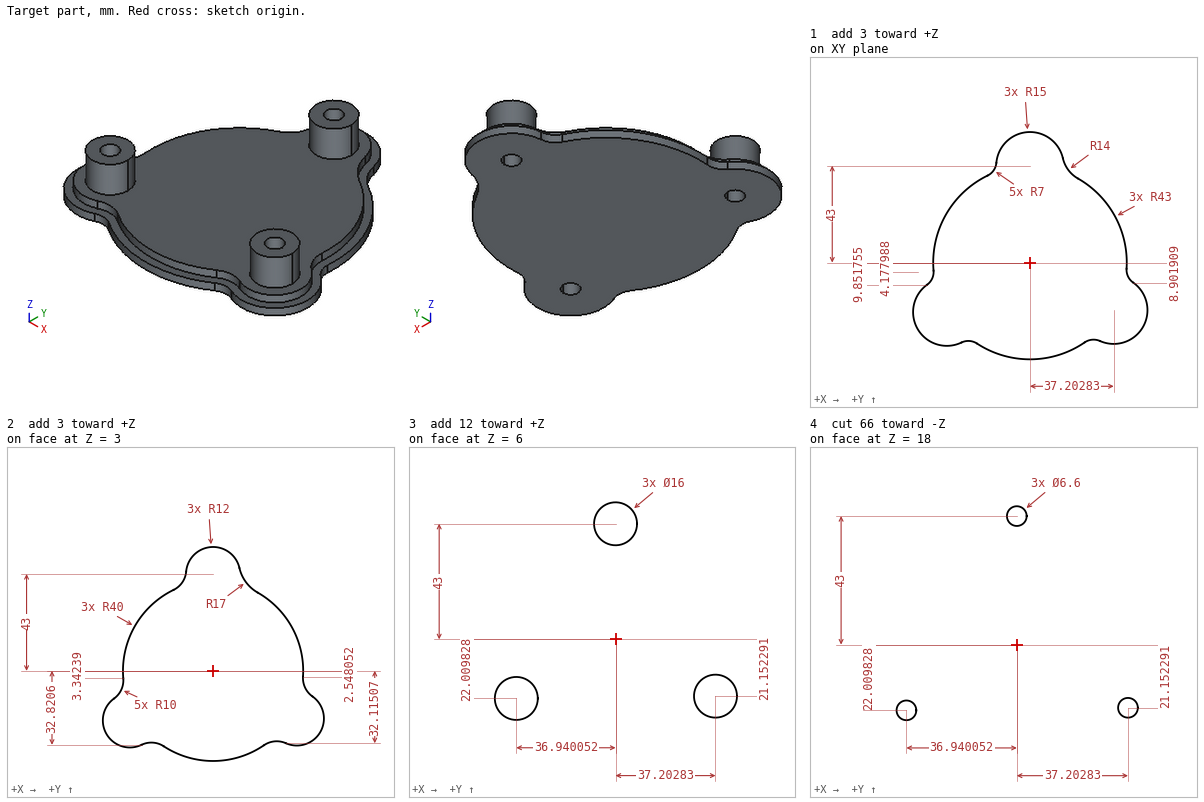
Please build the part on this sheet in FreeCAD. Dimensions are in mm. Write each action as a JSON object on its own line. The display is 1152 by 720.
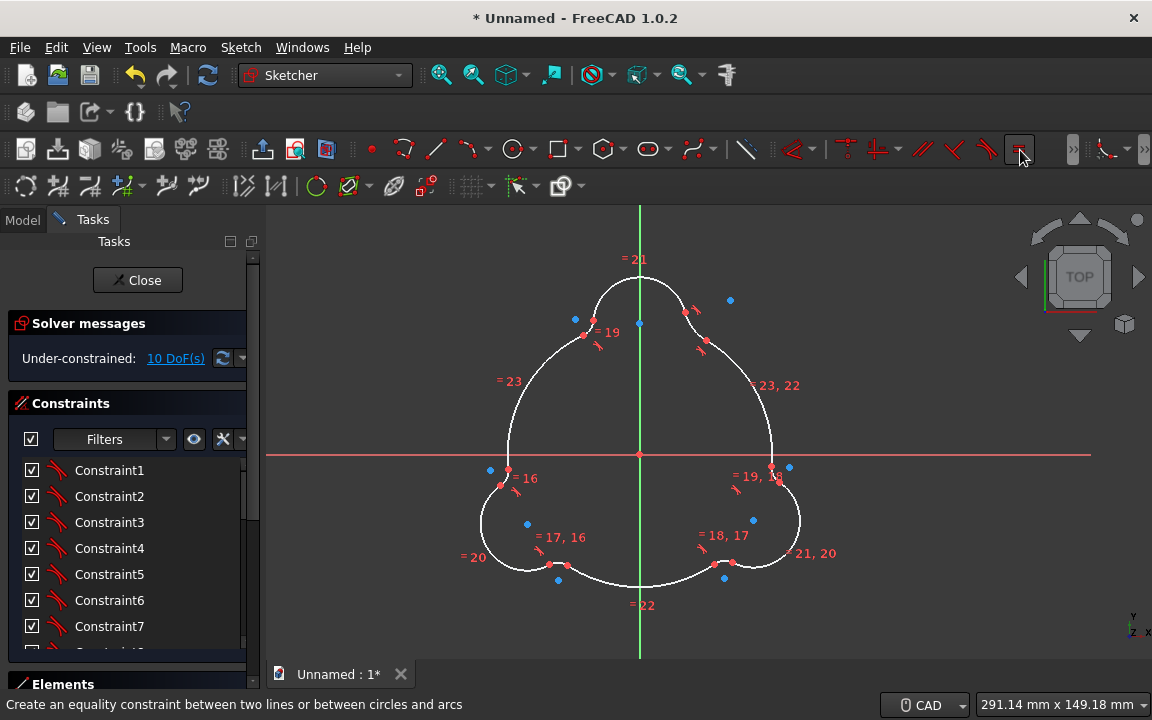
{"action": "left_click", "coordinate": [640, 324]}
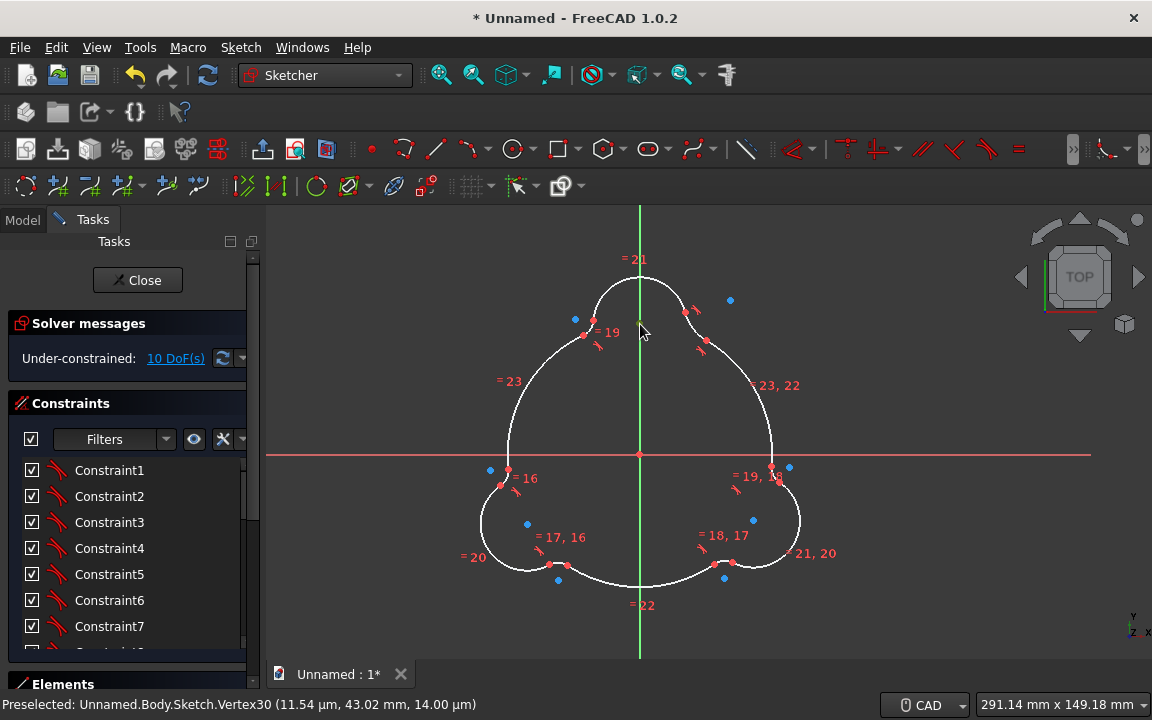
{"action": "left_click", "coordinate": [640, 546]}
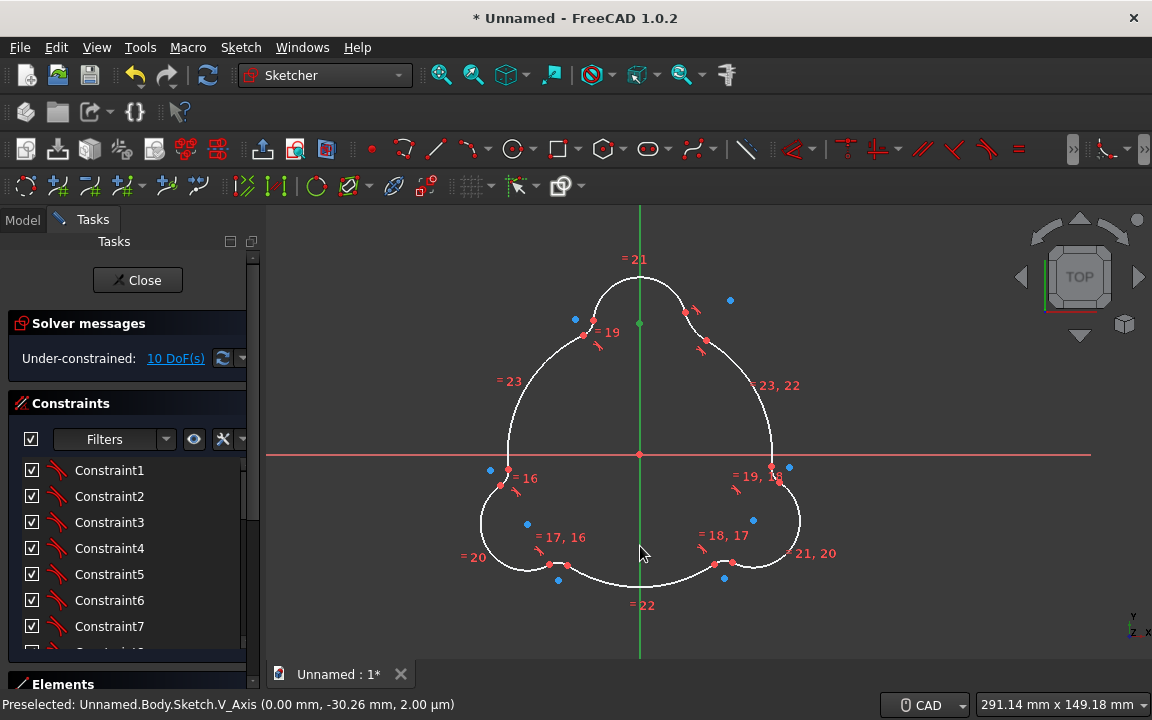
{"action": "left_click", "coordinate": [846, 150]}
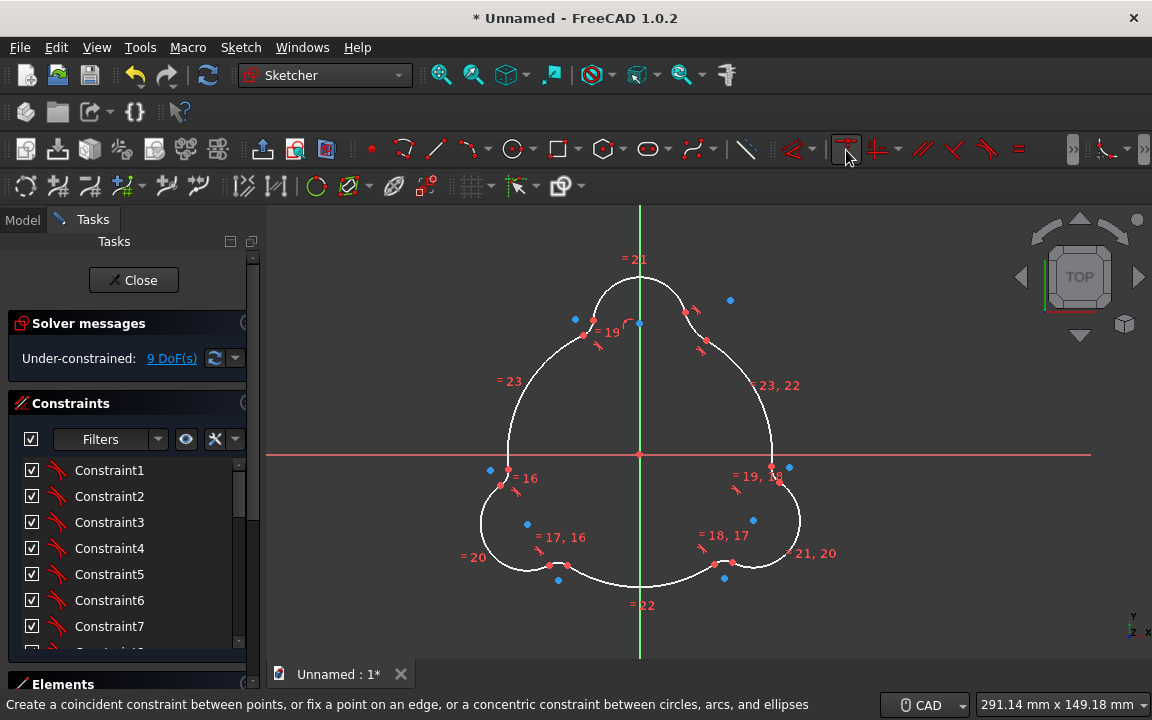
{"action": "left_click", "coordinate": [792, 150]}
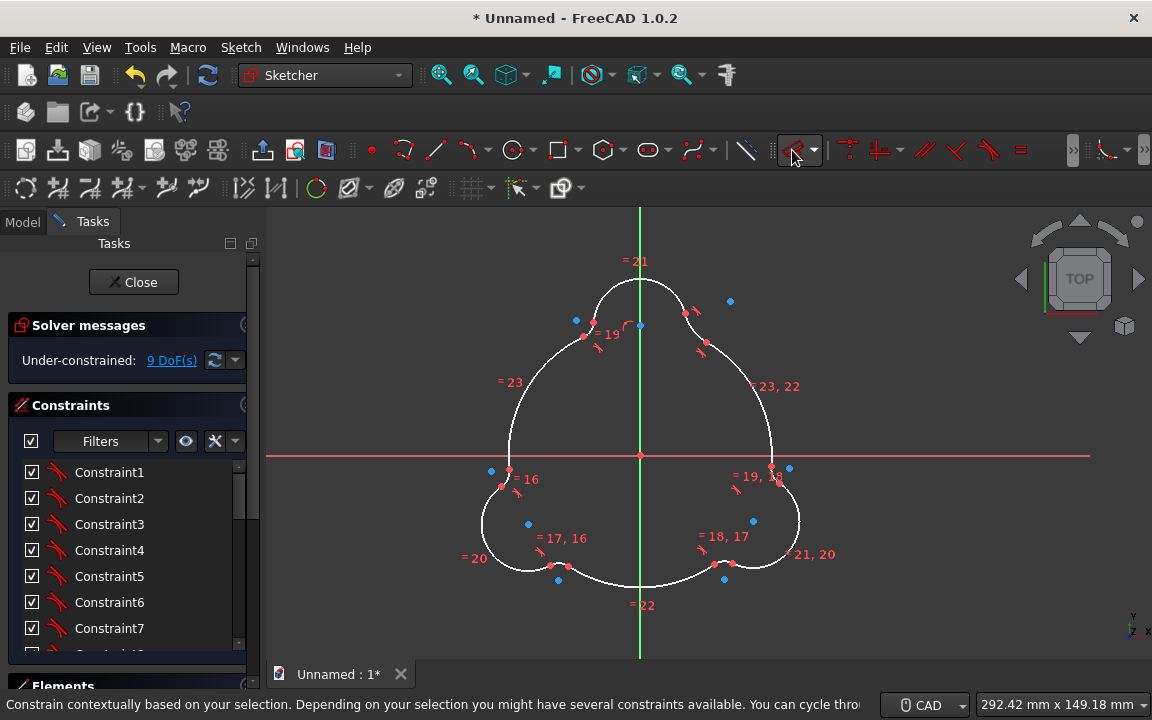
{"action": "scroll", "coordinate": [508, 479], "scroll_direction": "up", "scroll_amount": 4}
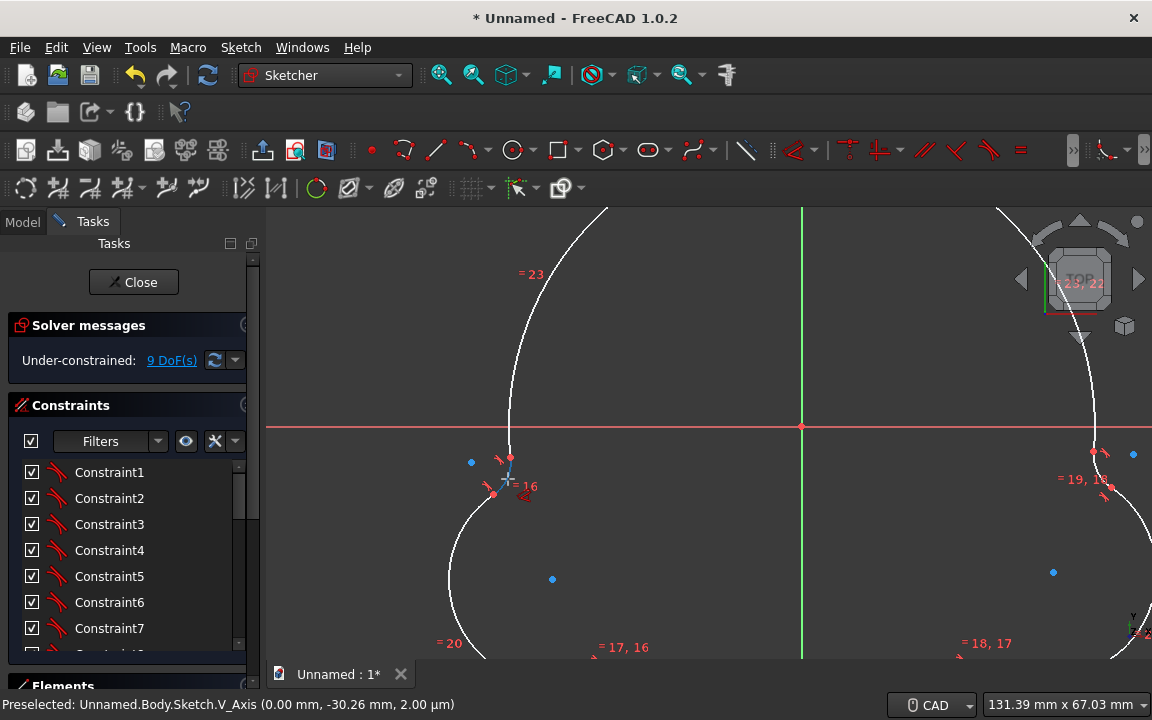
{"action": "left_click", "coordinate": [507, 479]}
{"action": "left_click", "coordinate": [536, 493]}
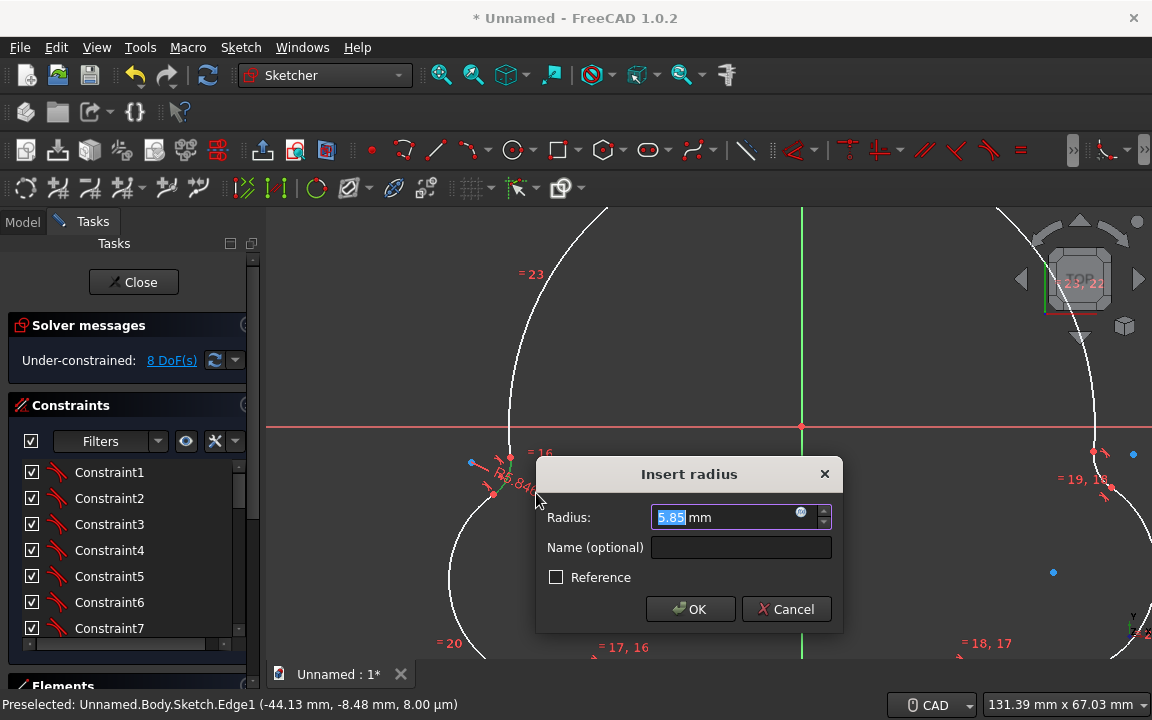
{"action": "type", "text": "7"}
{"action": "key", "text": "Return"}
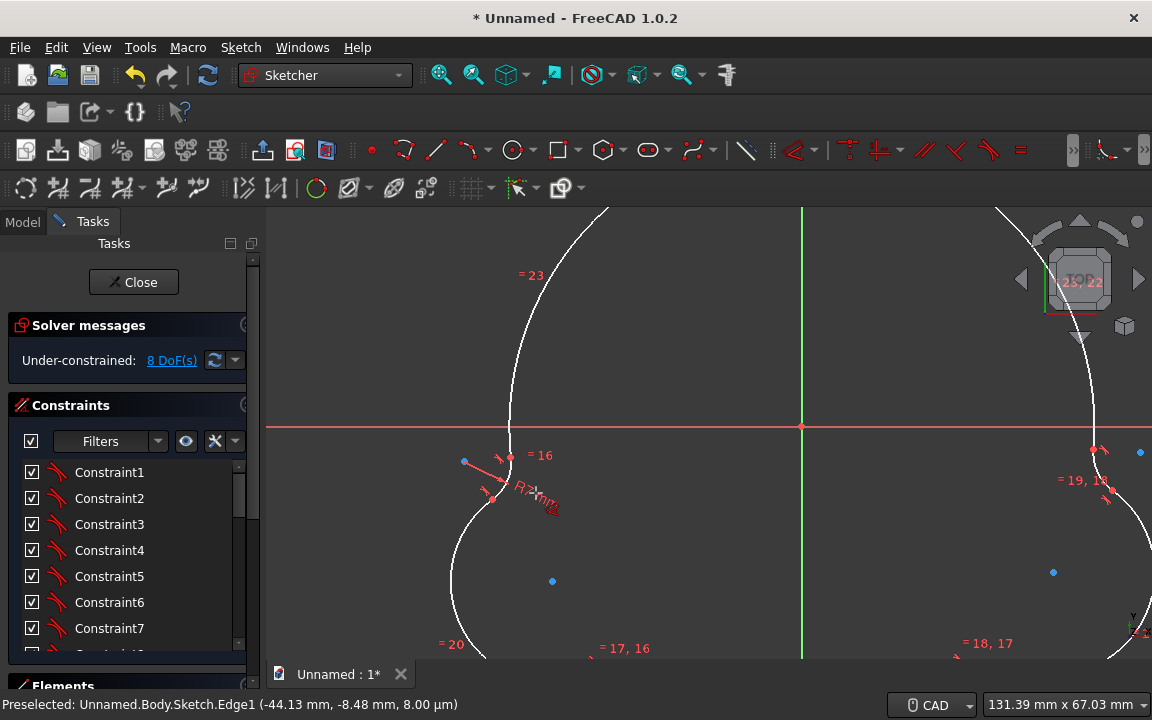
{"action": "left_click", "coordinate": [451, 578]}
{"action": "left_click", "coordinate": [419, 577]}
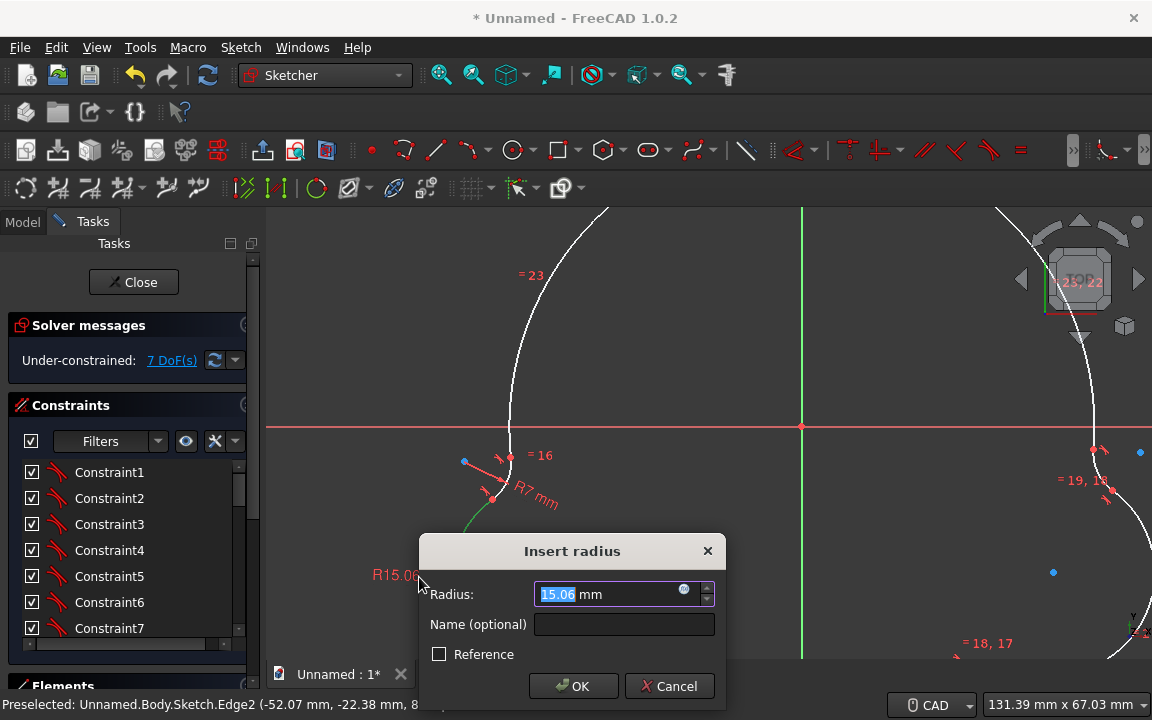
{"action": "type", "text": "15"}
{"action": "key", "text": "Return"}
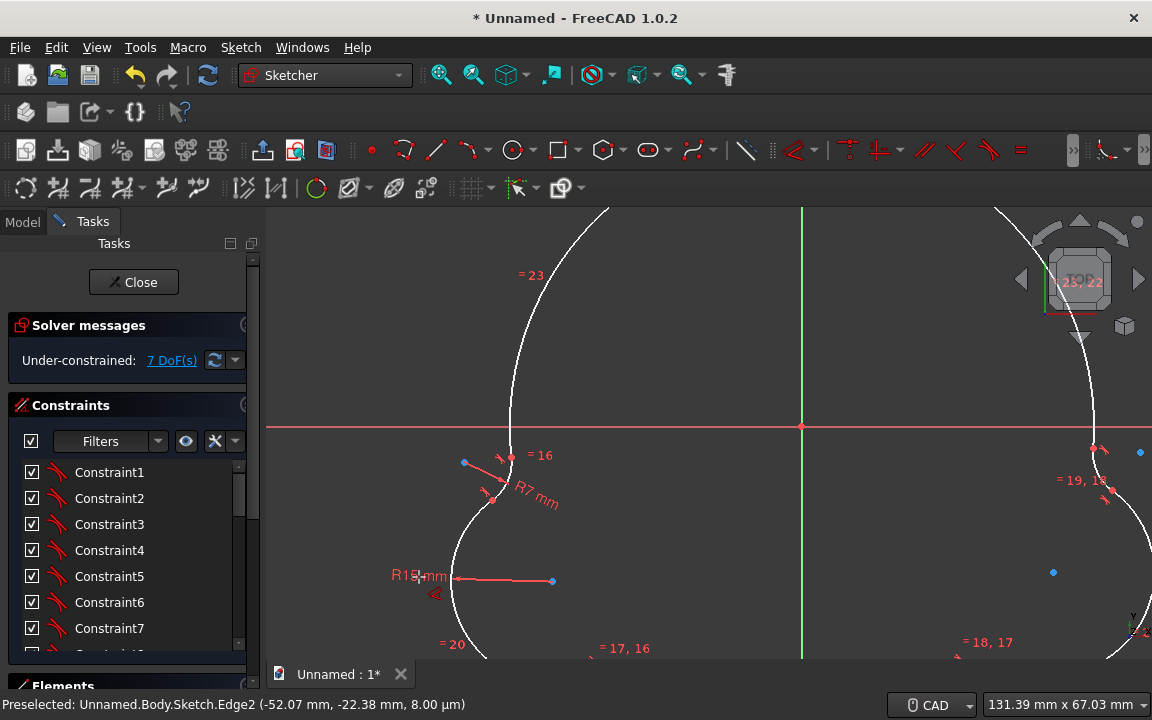
{"action": "scroll", "coordinate": [508, 479], "scroll_direction": "down", "scroll_amount": 4}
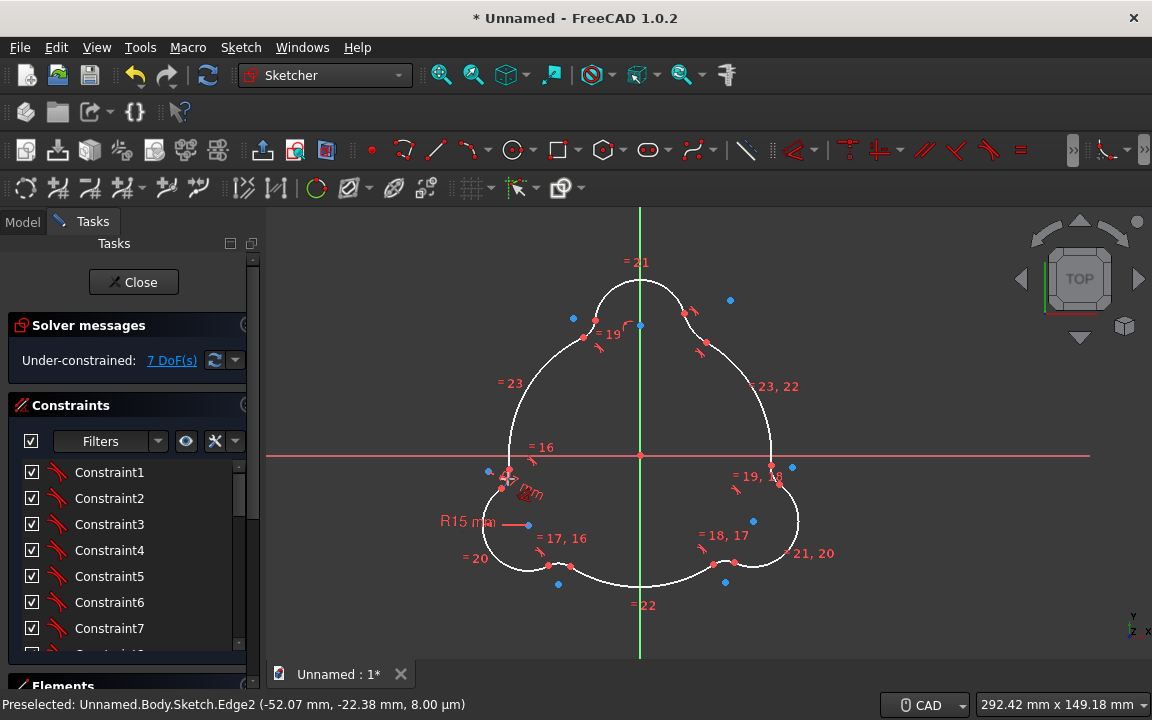
{"action": "left_click", "coordinate": [612, 584]}
{"action": "left_click", "coordinate": [605, 615]}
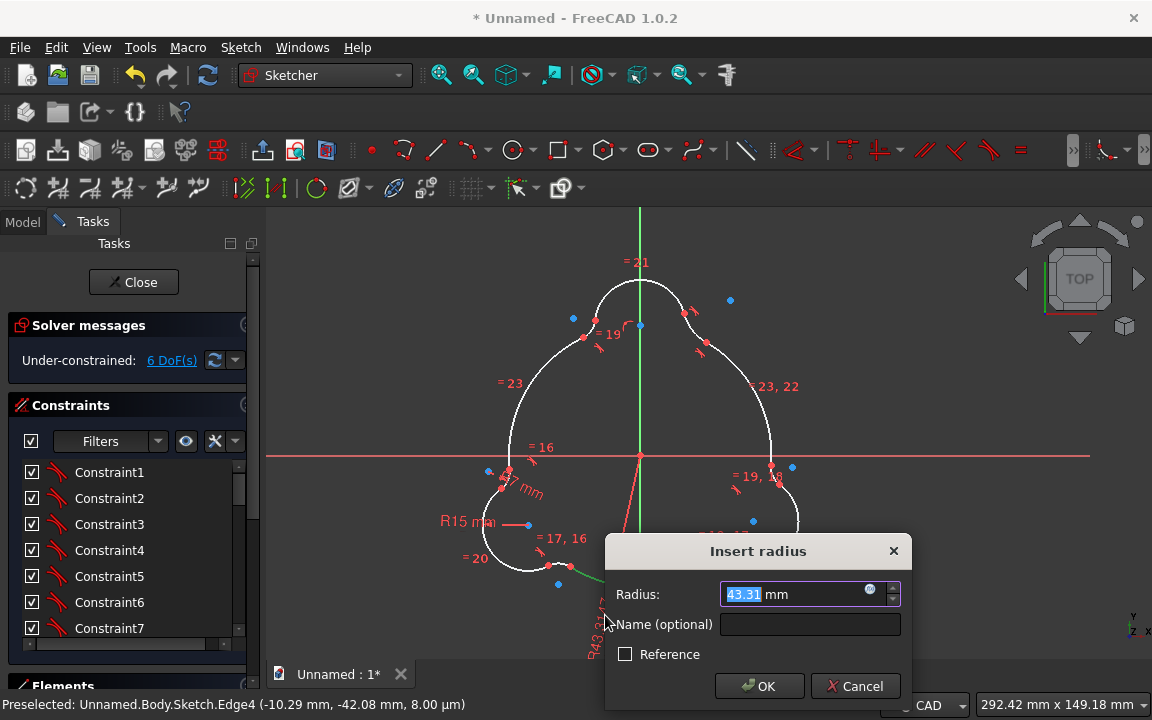
{"action": "type", "text": "43"}
{"action": "key", "text": "Return"}